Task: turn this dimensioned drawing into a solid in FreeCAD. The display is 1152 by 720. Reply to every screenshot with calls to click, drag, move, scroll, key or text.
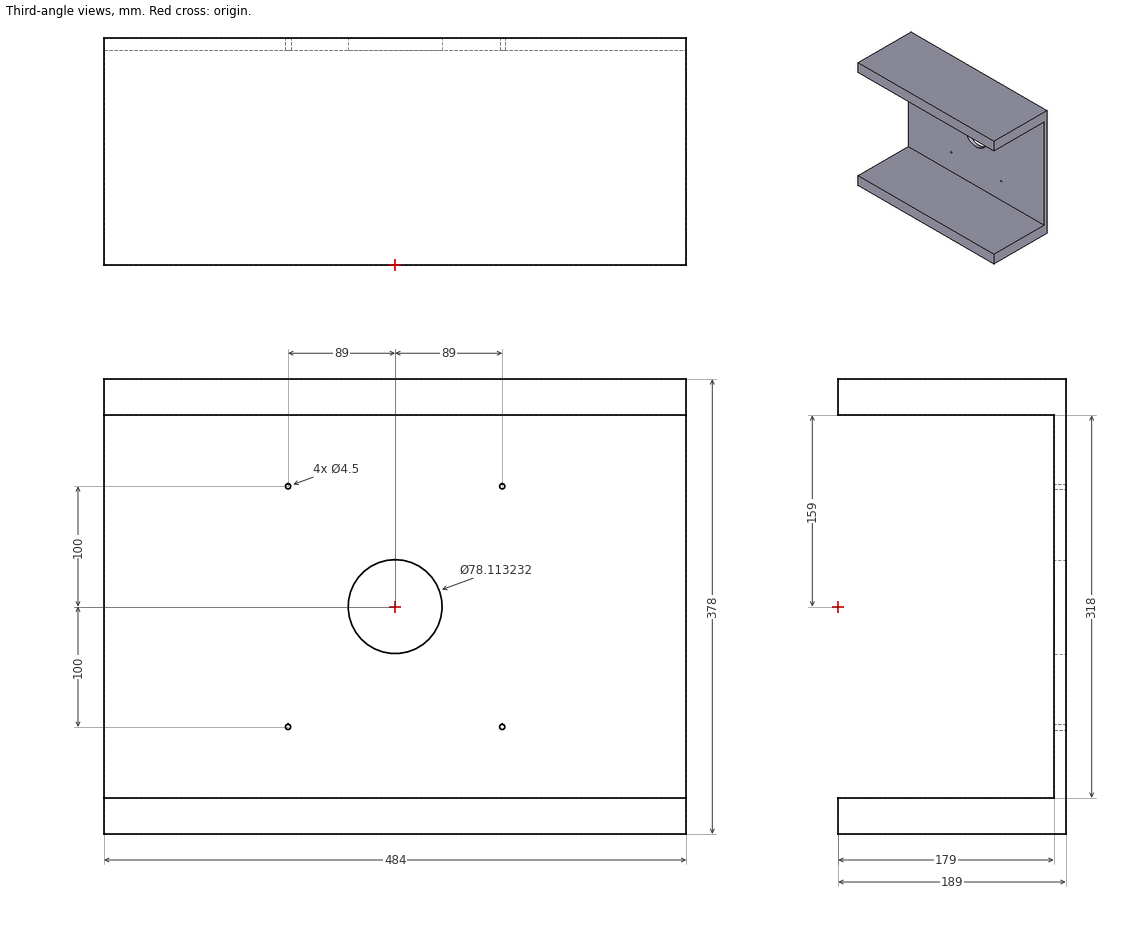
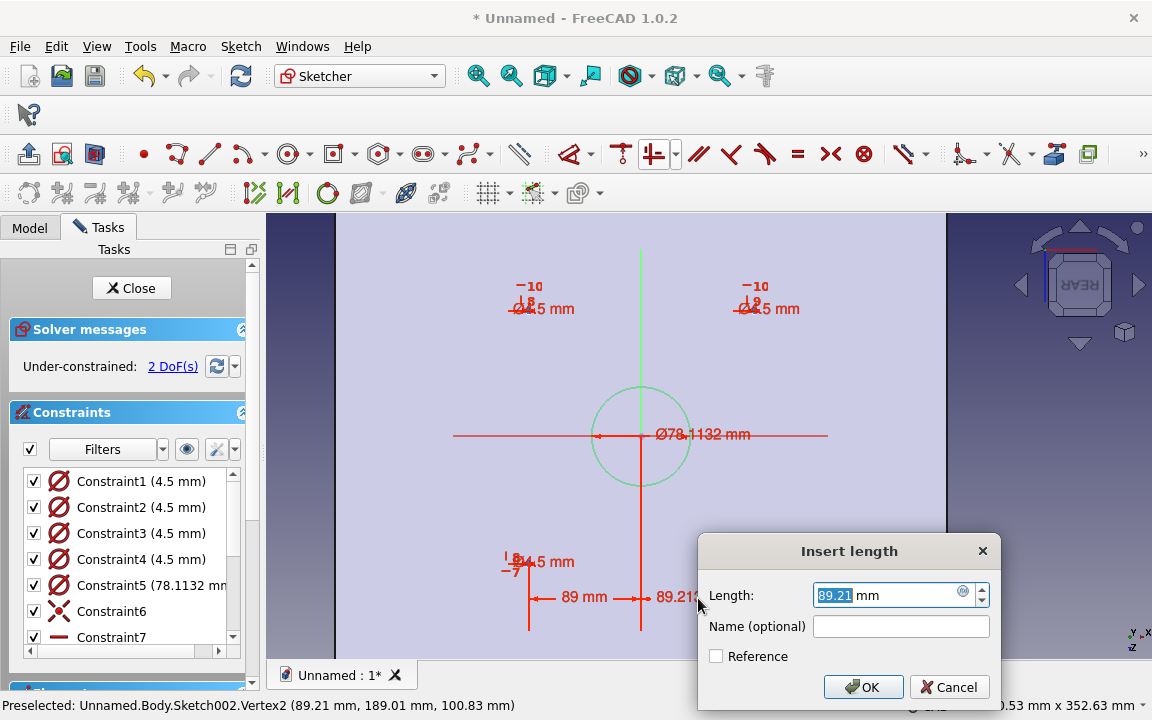
text(89)
key(Return)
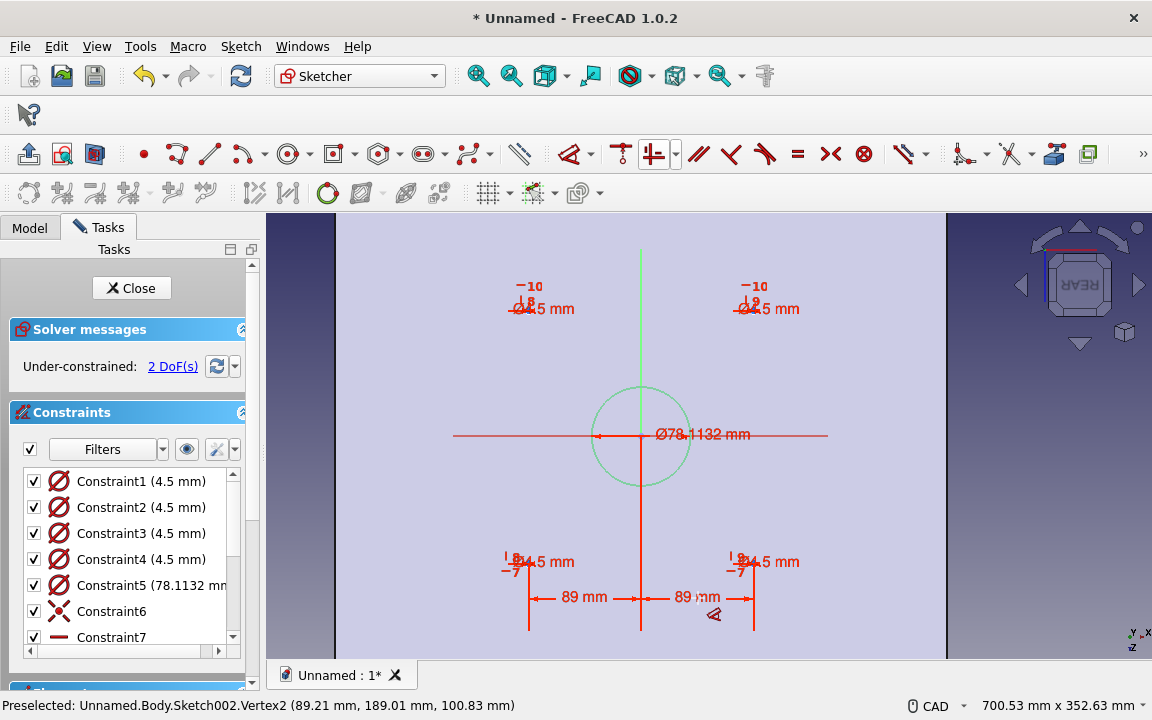
click(529, 564)
click(495, 500)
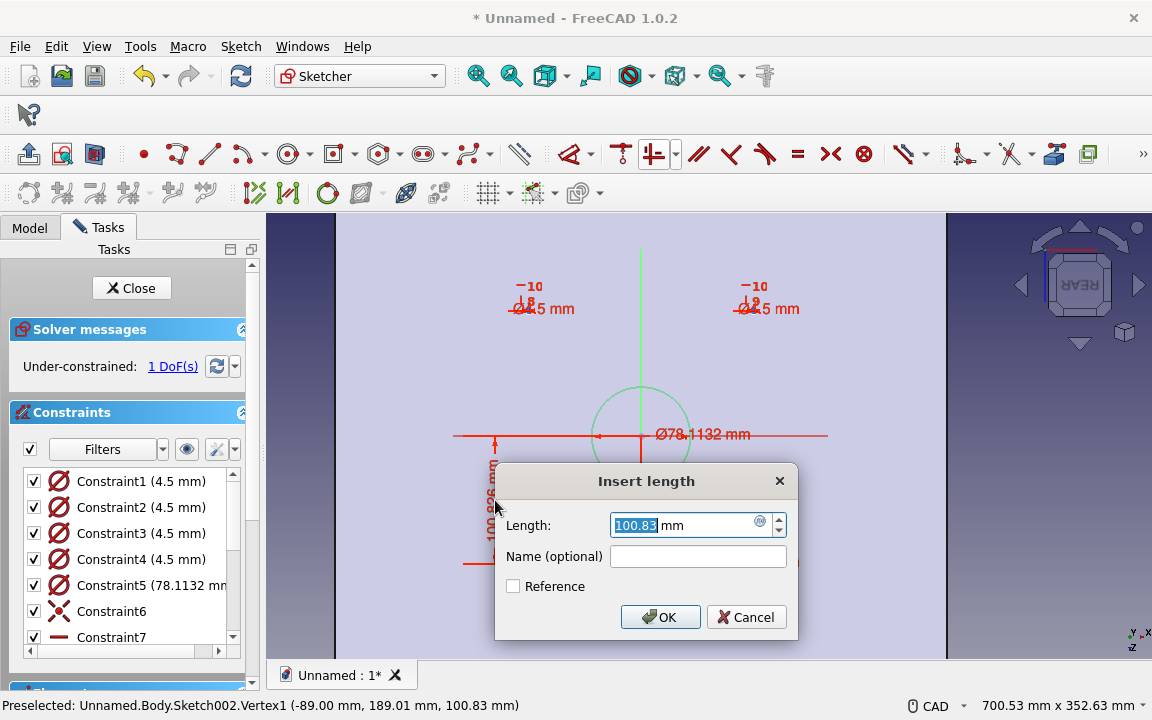
text(100)
key(Return)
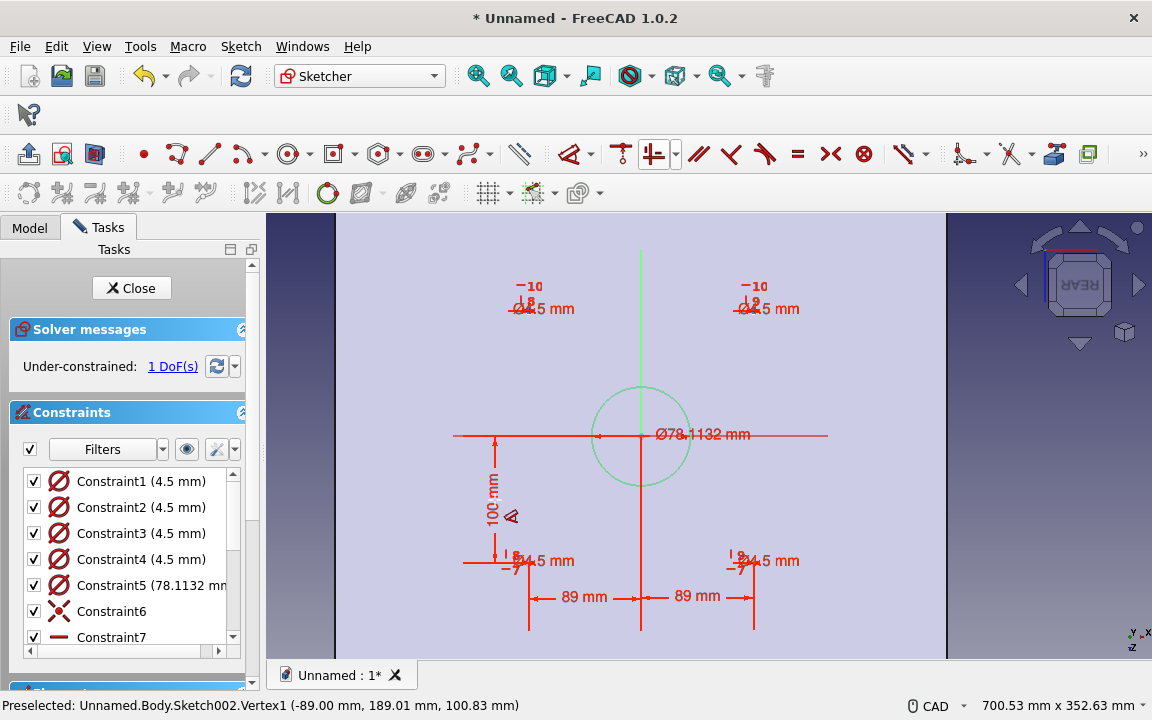
click(529, 311)
click(495, 374)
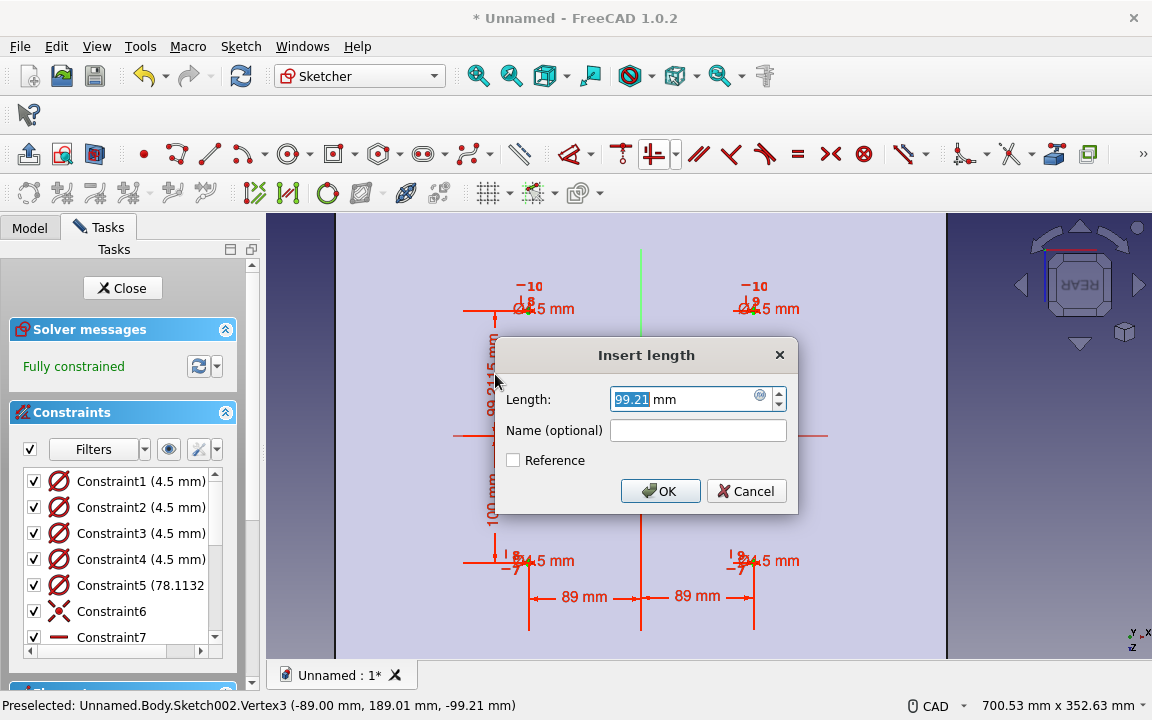
text(100)
key(Return)
key(Escape)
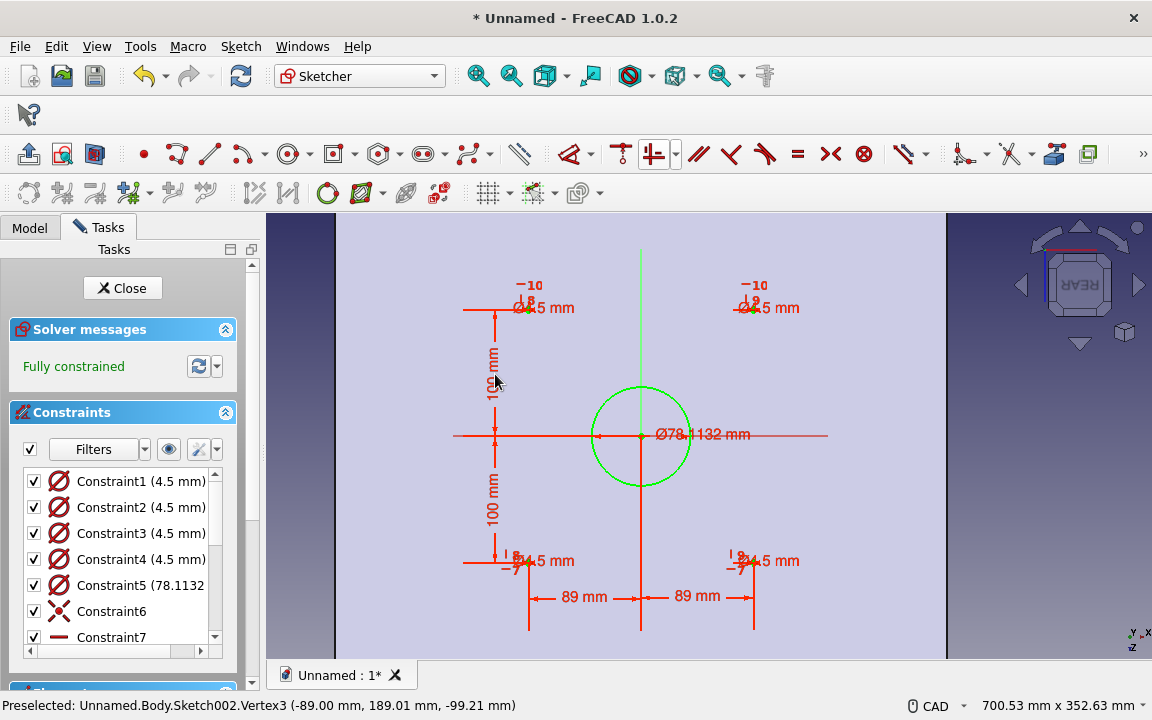
click(123, 288)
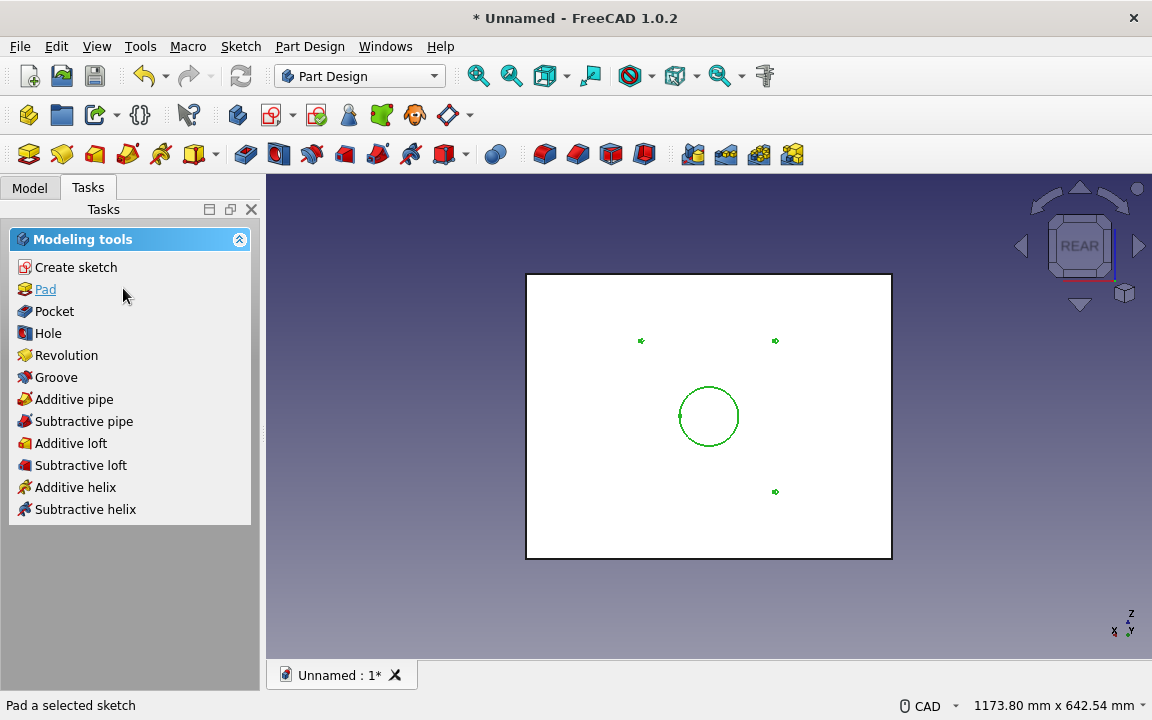
click(246, 154)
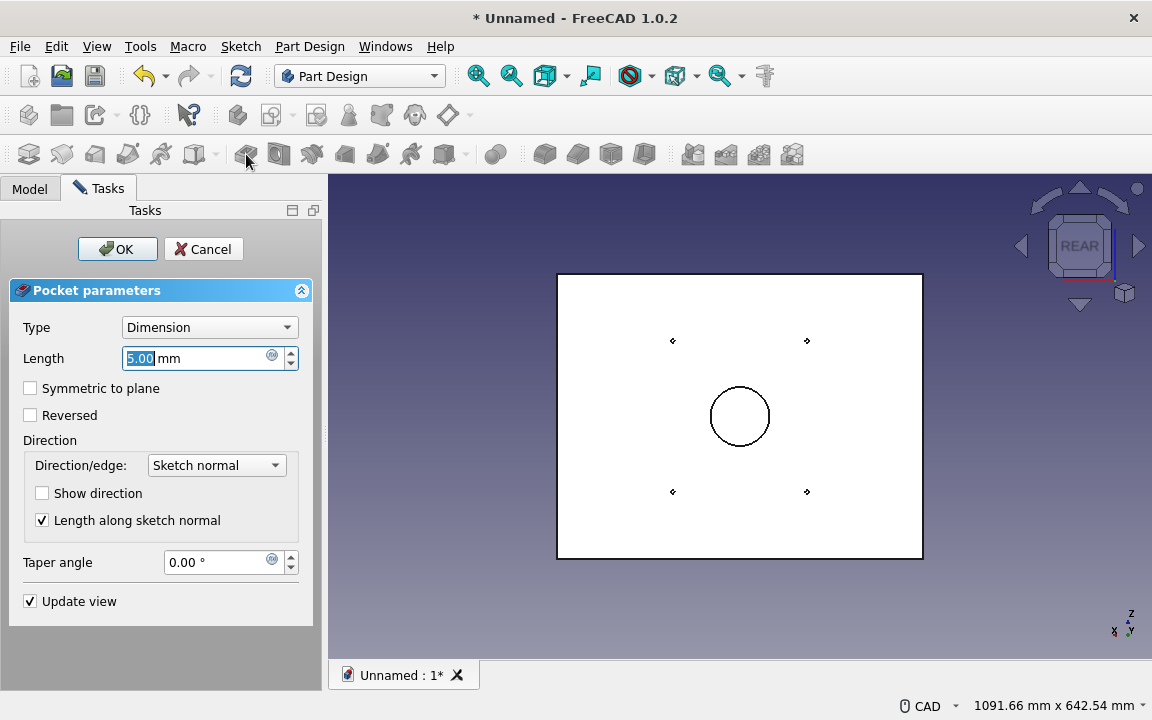
click(210, 328)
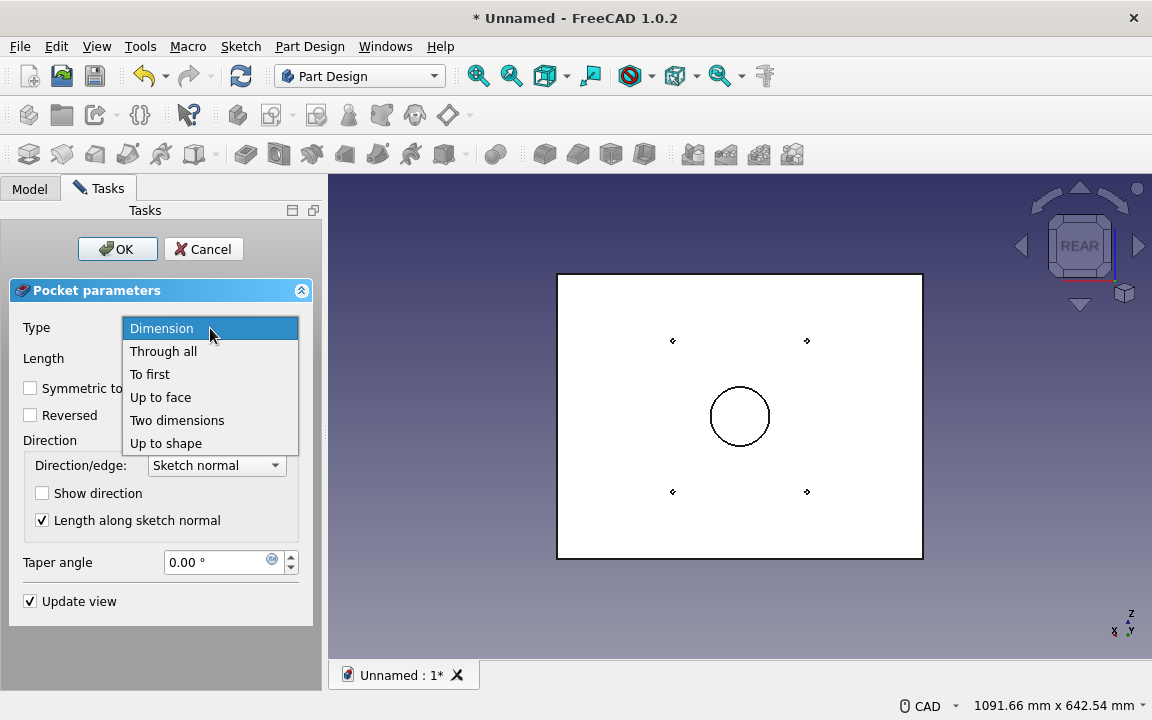
click(208, 352)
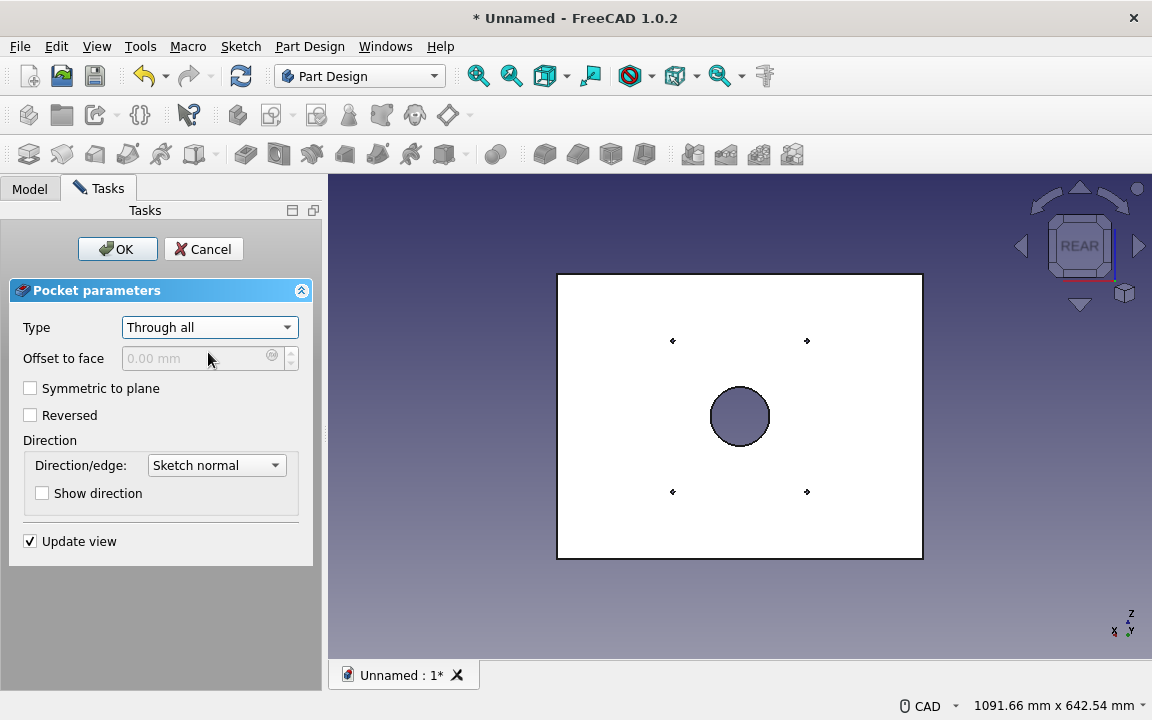
click(118, 249)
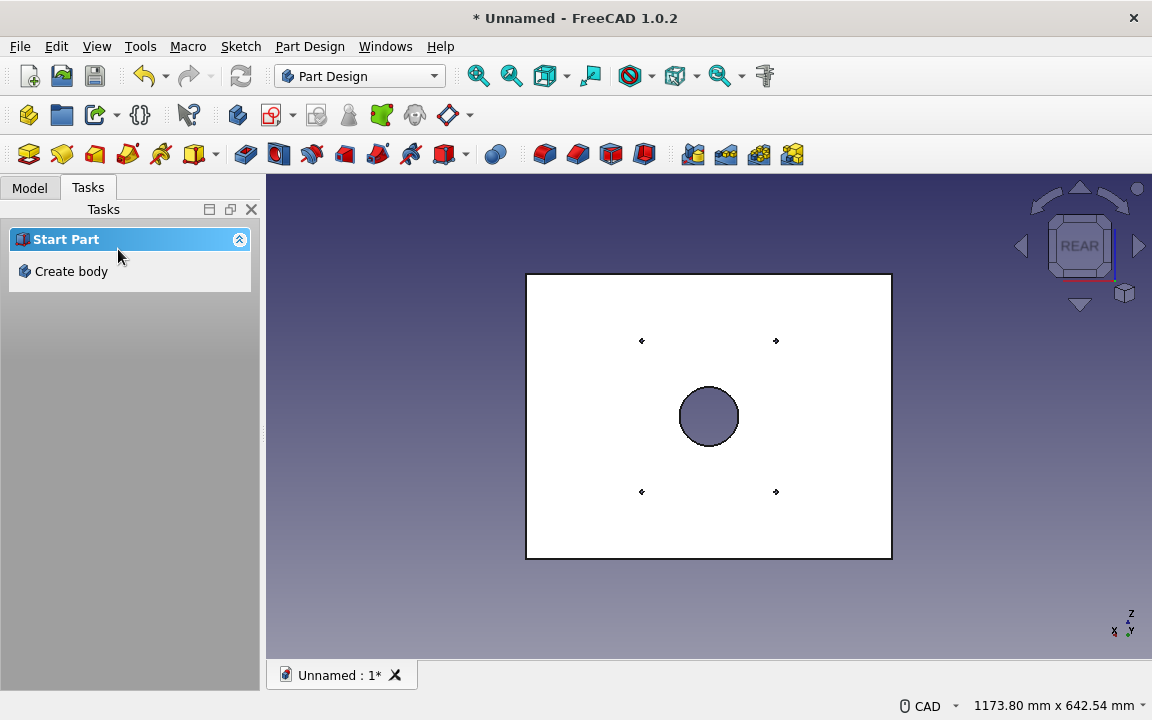
key(0)